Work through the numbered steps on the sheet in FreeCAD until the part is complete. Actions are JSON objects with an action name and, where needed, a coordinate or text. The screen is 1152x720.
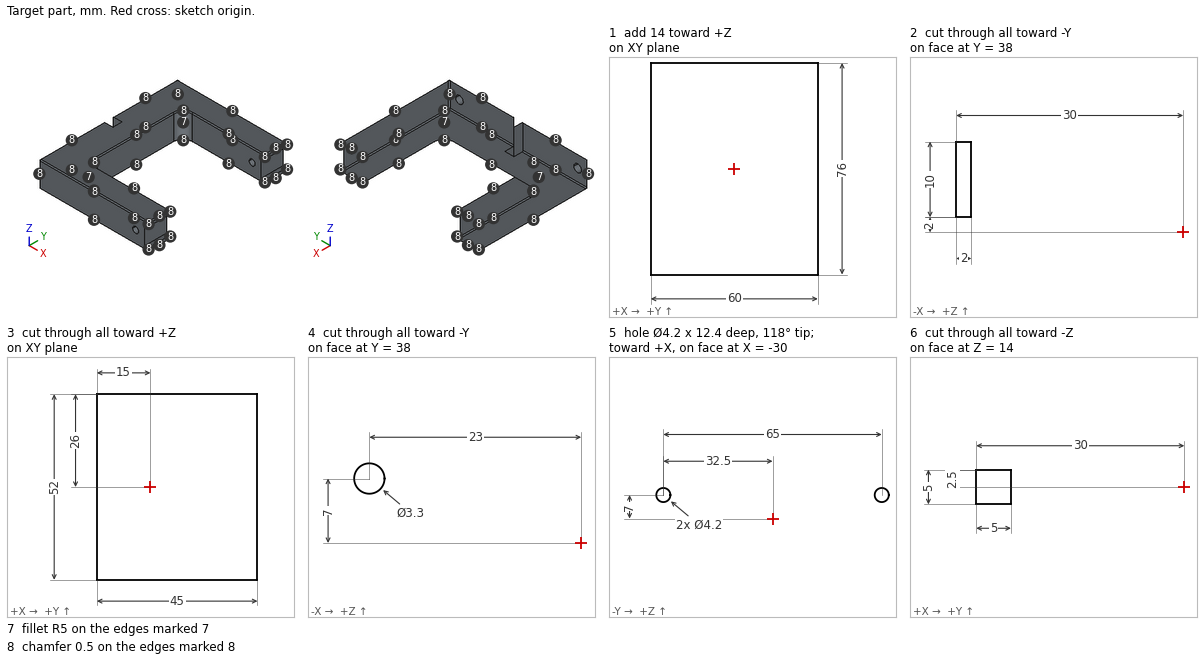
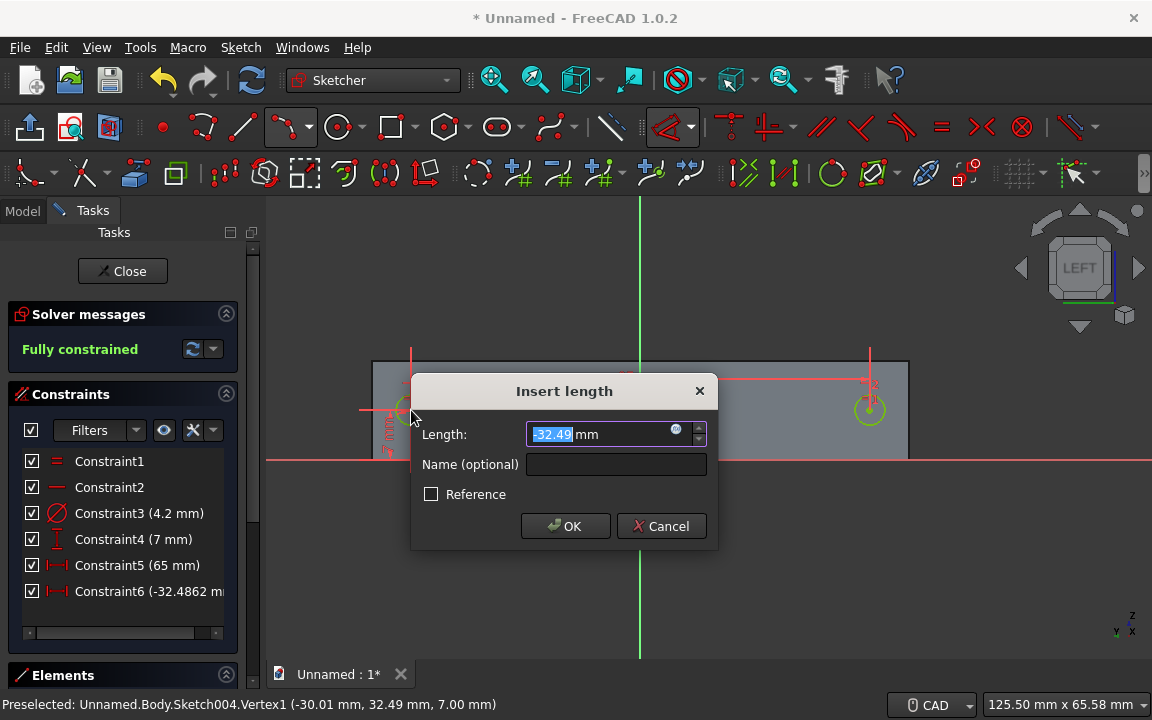
{"action": "type", "text": "-32.5"}
{"action": "key", "text": "Return"}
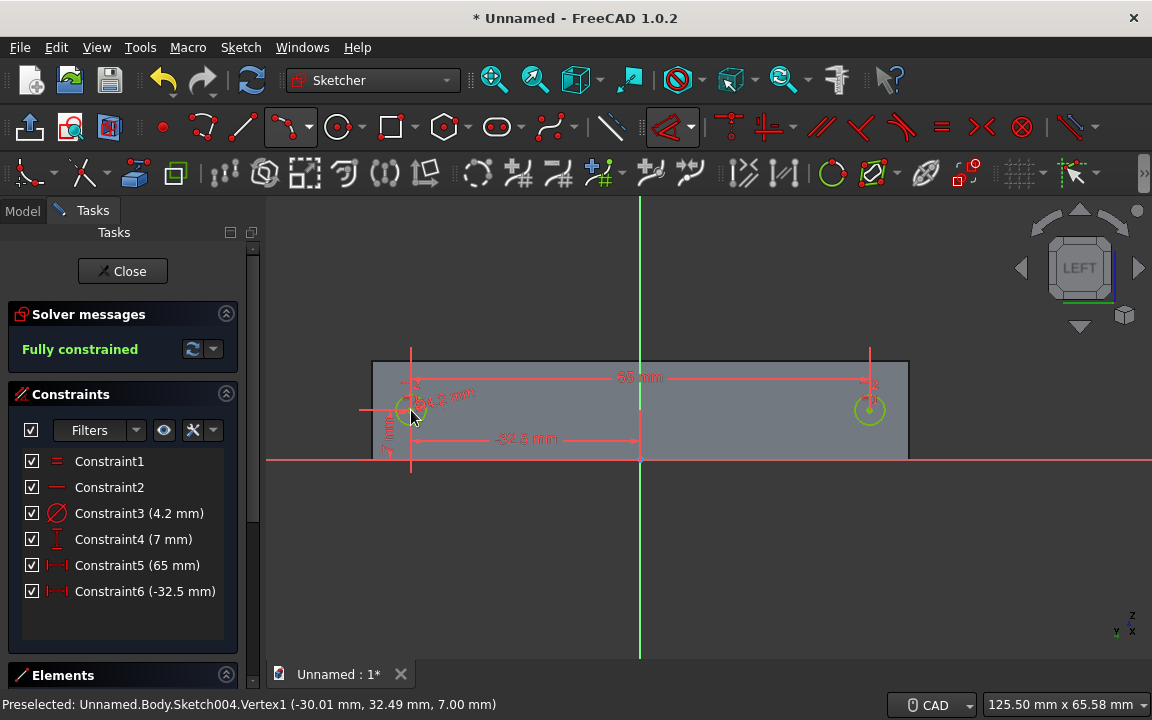
{"action": "left_click", "coordinate": [123, 271]}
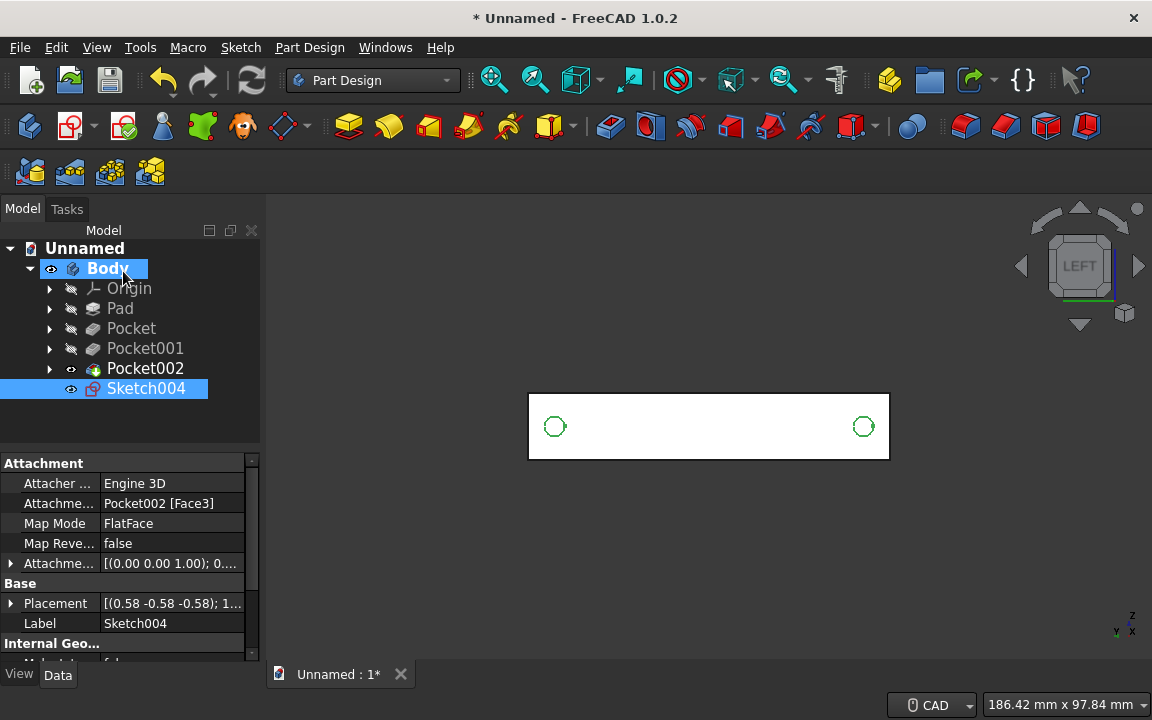
{"action": "left_click", "coordinate": [652, 126]}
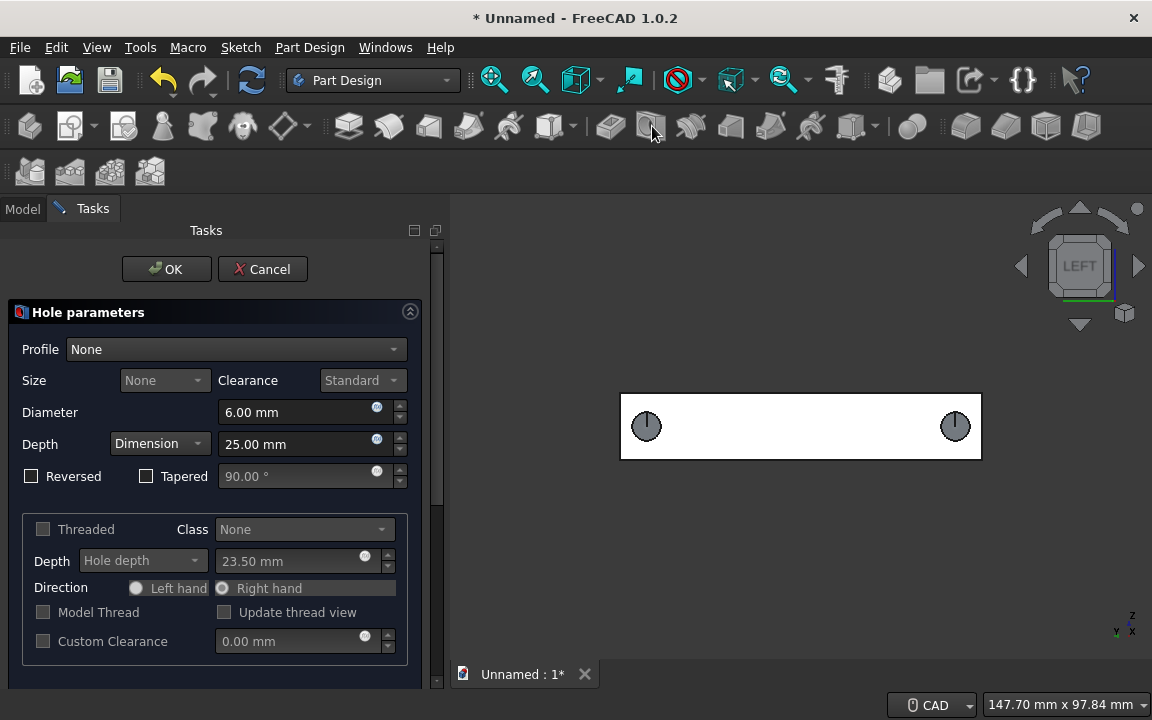
{"action": "triple_click", "coordinate": [305, 412]}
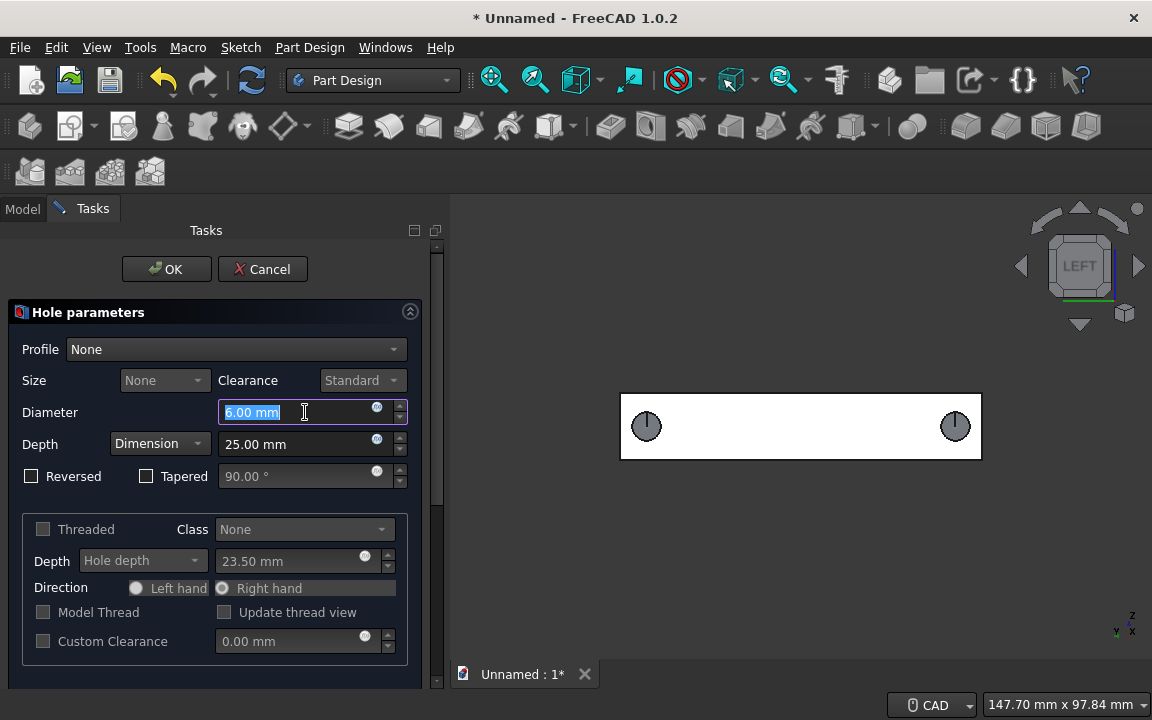
{"action": "type", "text": "4.2"}
{"action": "key", "text": "Tab"}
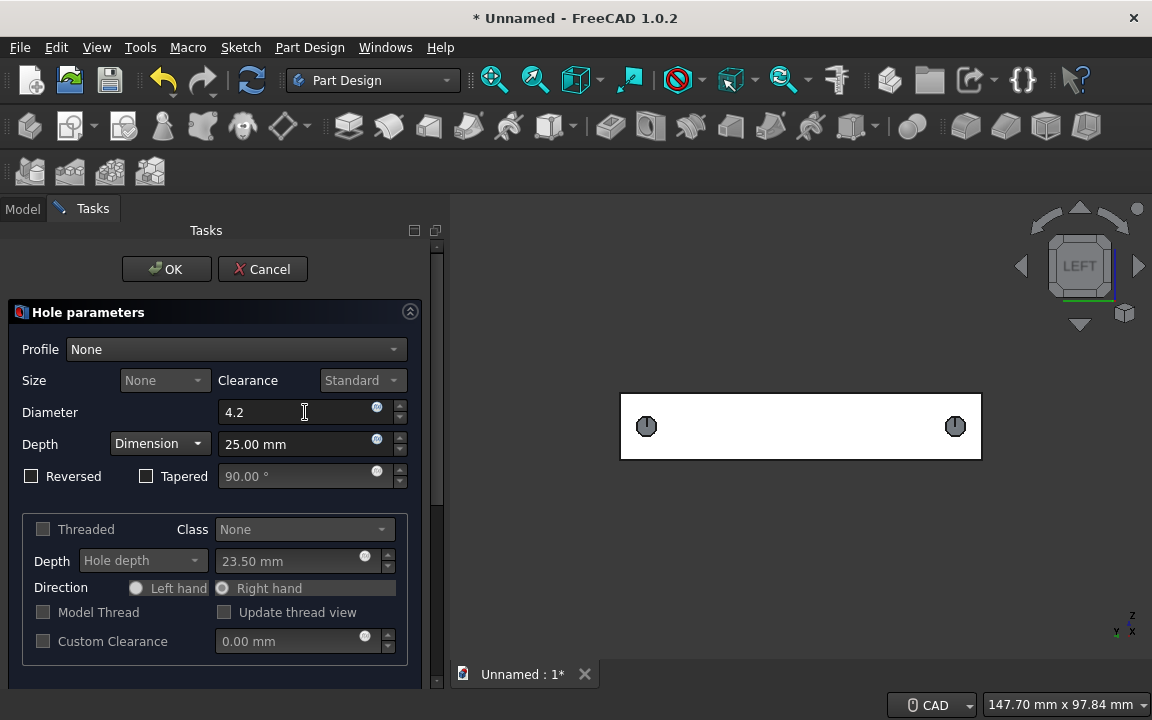
{"action": "triple_click", "coordinate": [305, 444]}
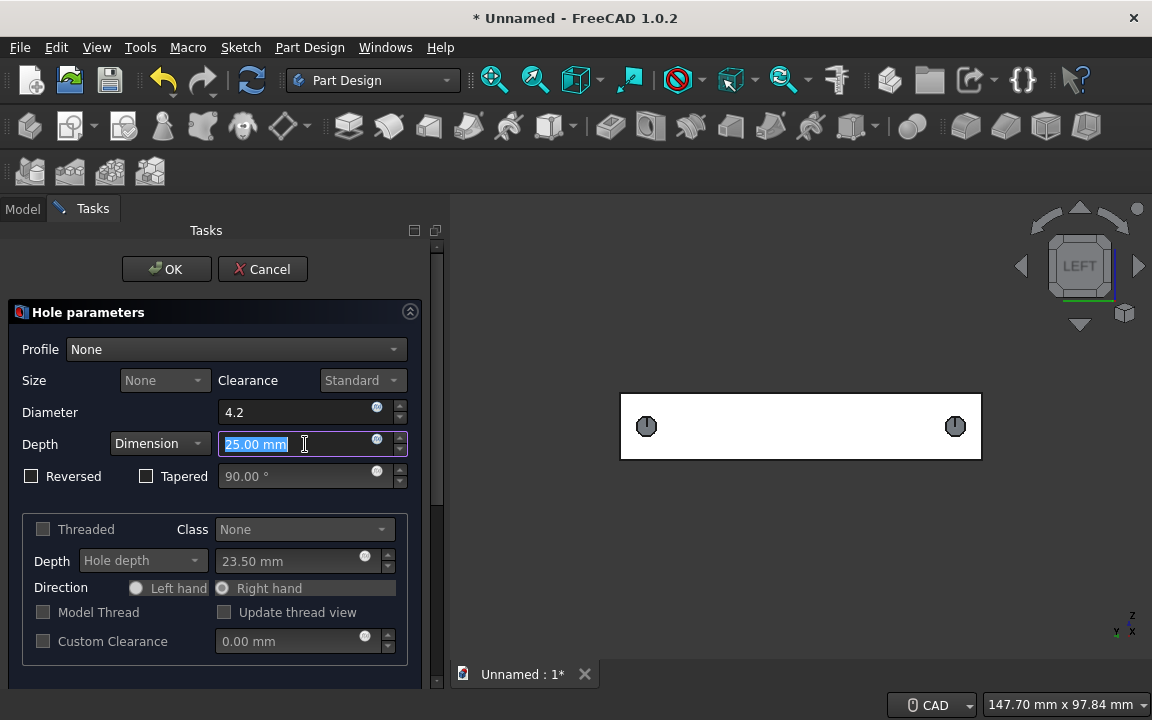
{"action": "type", "text": "12.4"}
{"action": "key", "text": "Tab"}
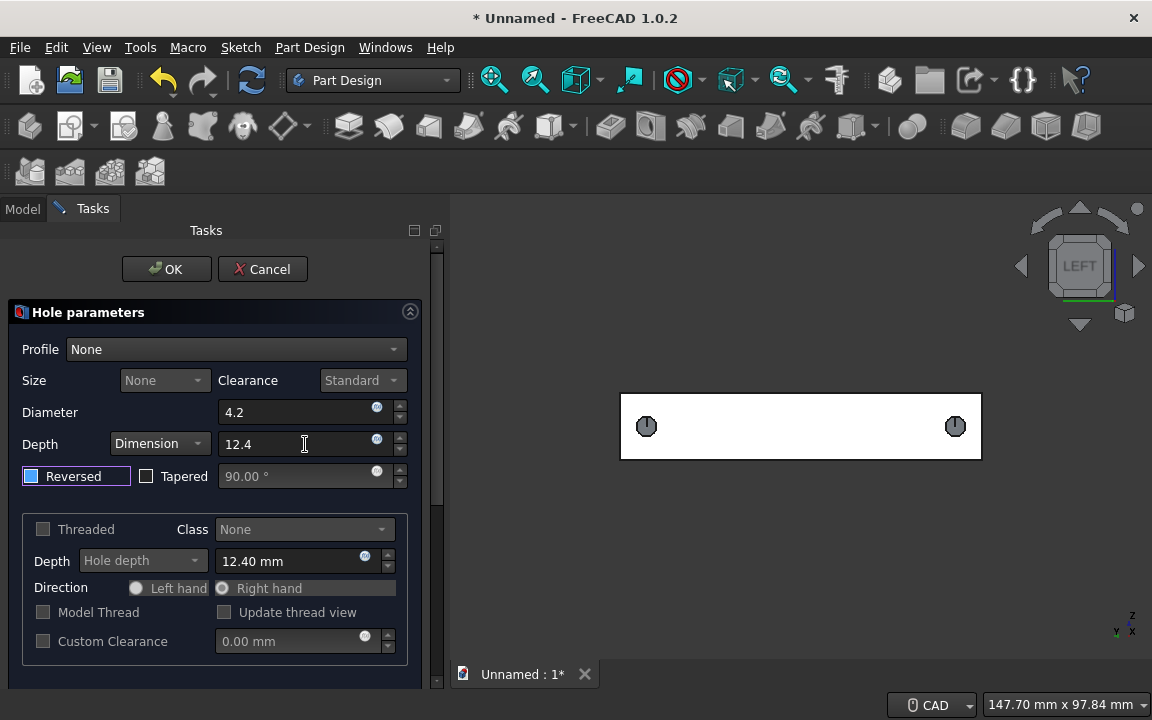
{"action": "left_click", "coordinate": [167, 269]}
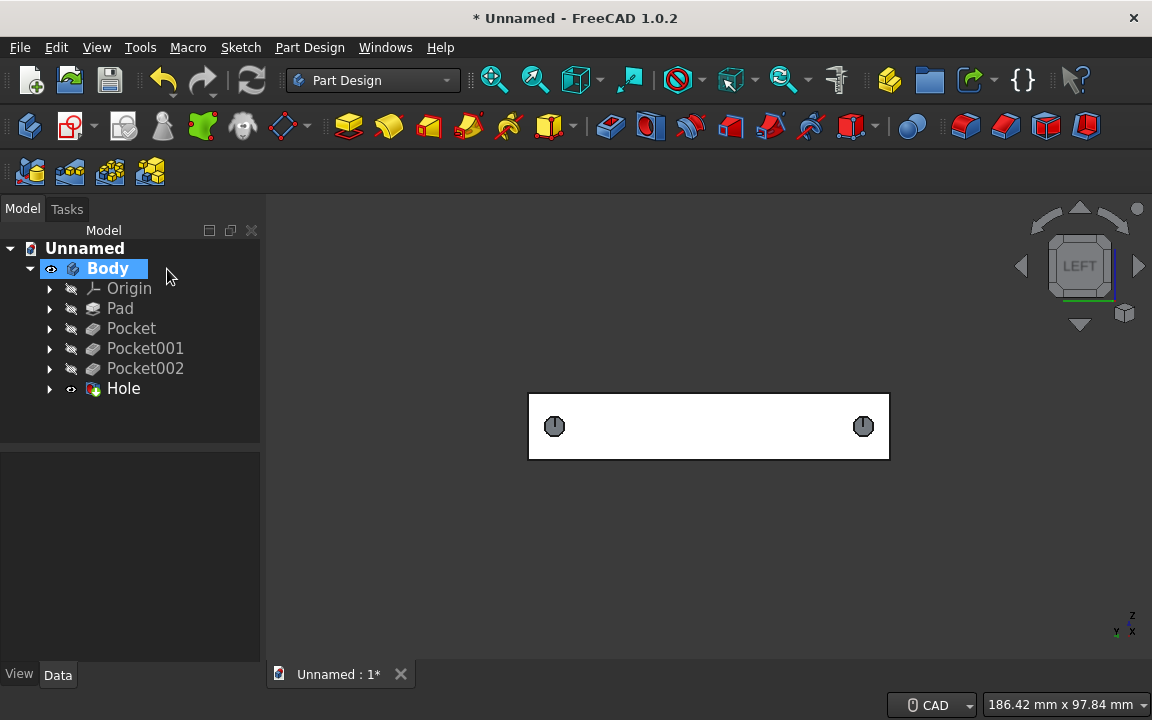
{"action": "key", "text": "v f"}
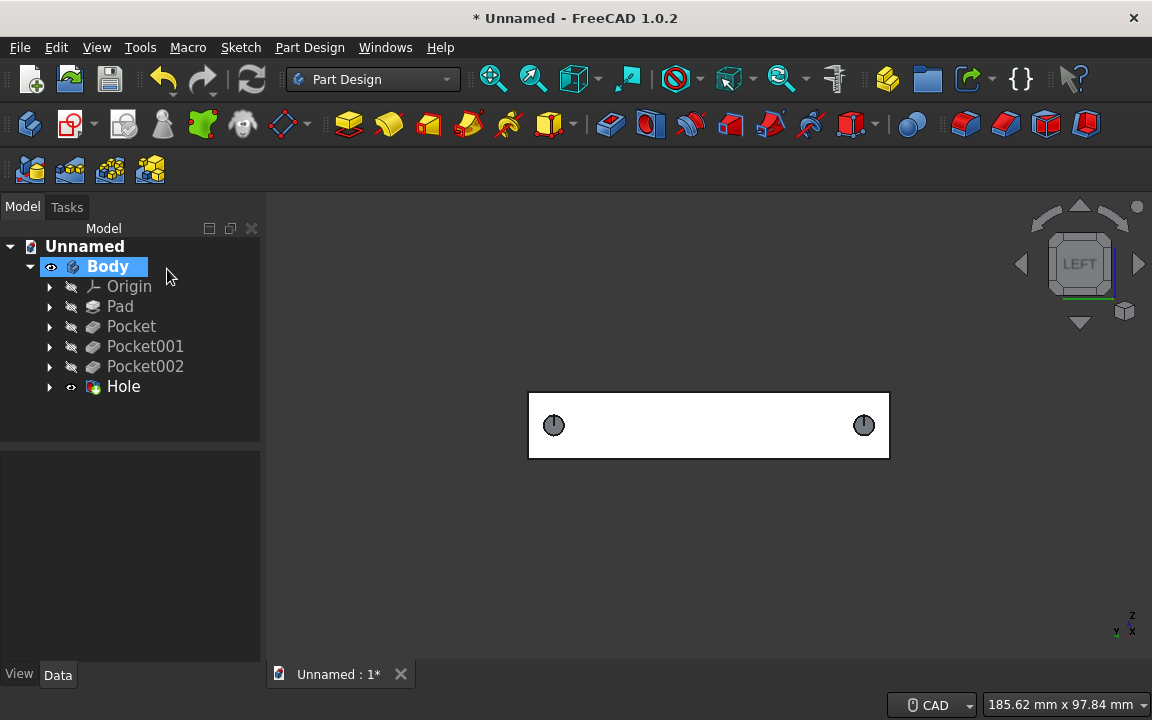
{"action": "key", "text": "0"}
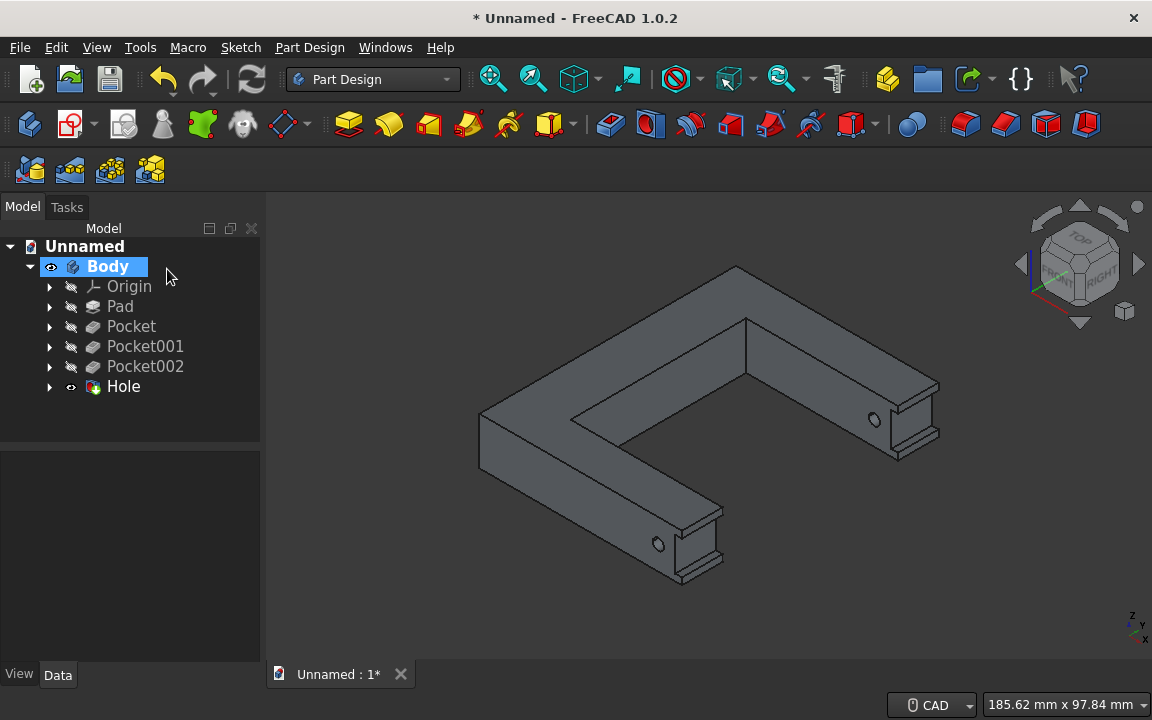
{"action": "left_click", "coordinate": [877, 367]}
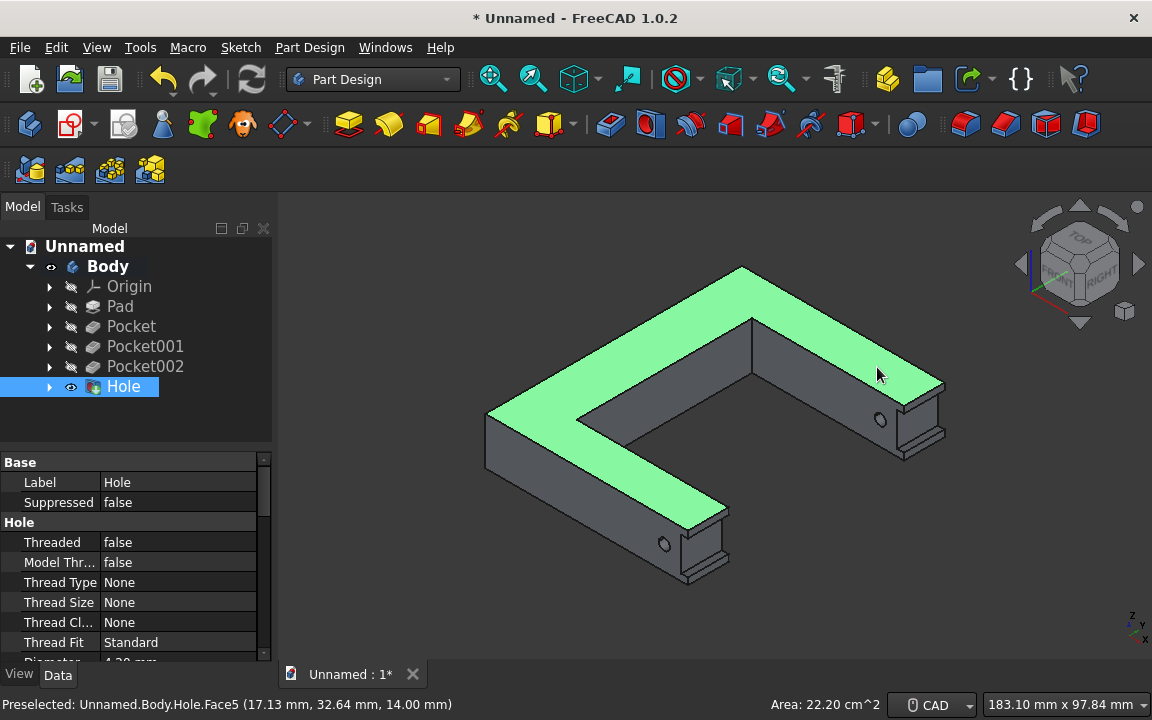
{"action": "left_click", "coordinate": [70, 124]}